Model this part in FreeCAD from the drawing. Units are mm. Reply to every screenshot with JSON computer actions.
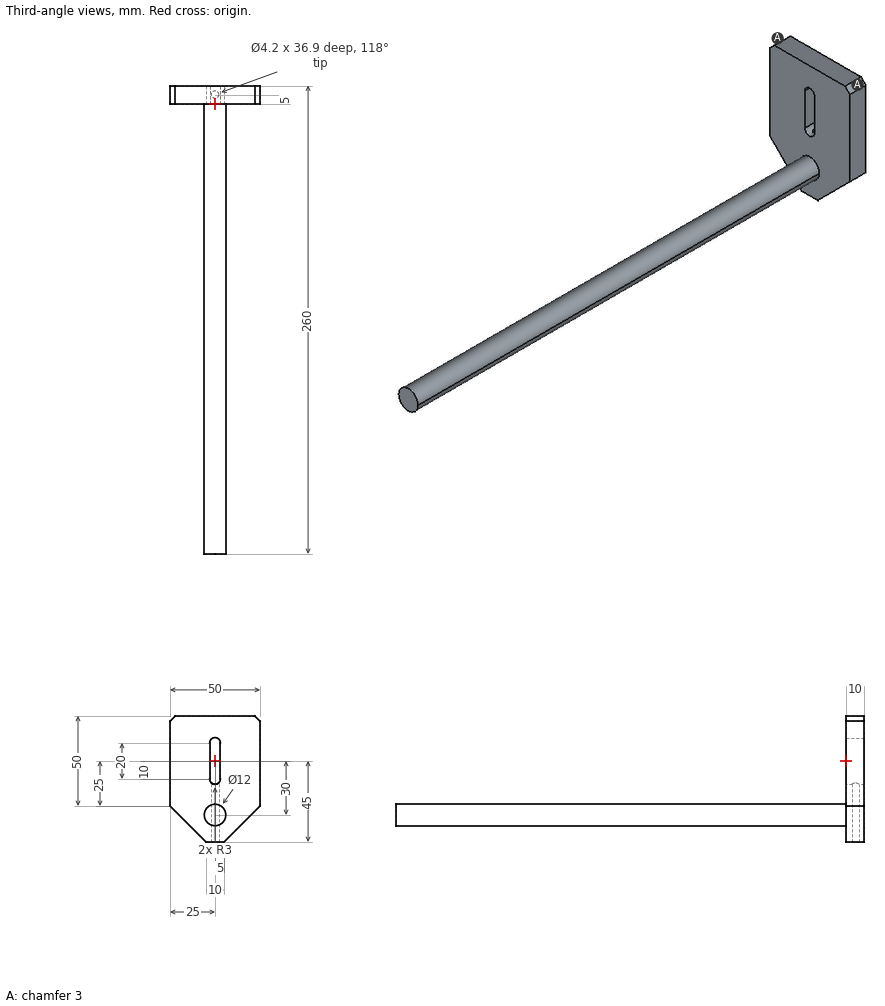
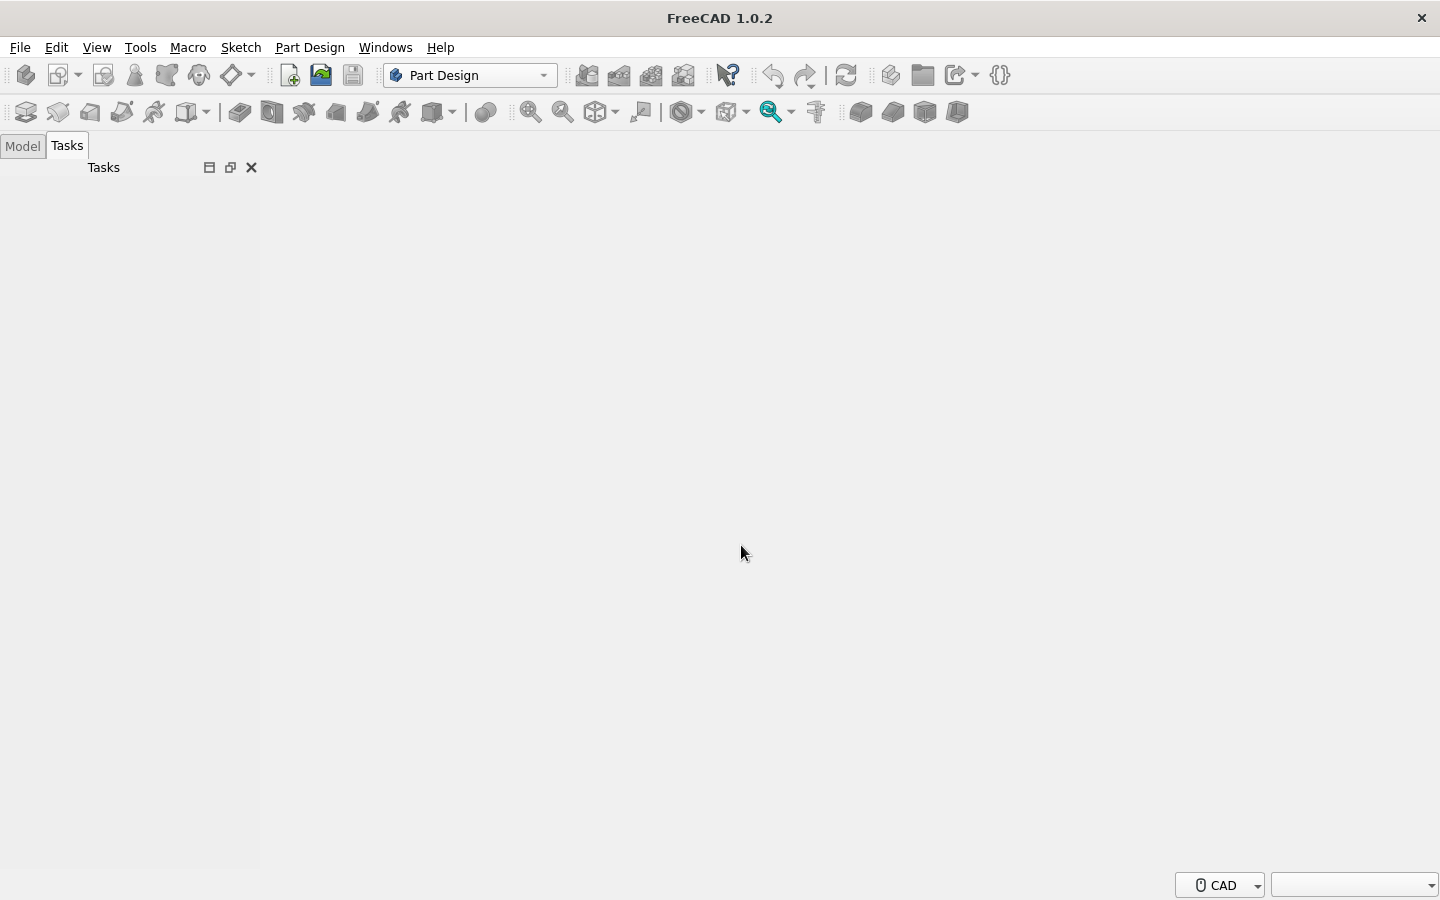
{"action": "left_click", "coordinate": [290, 76]}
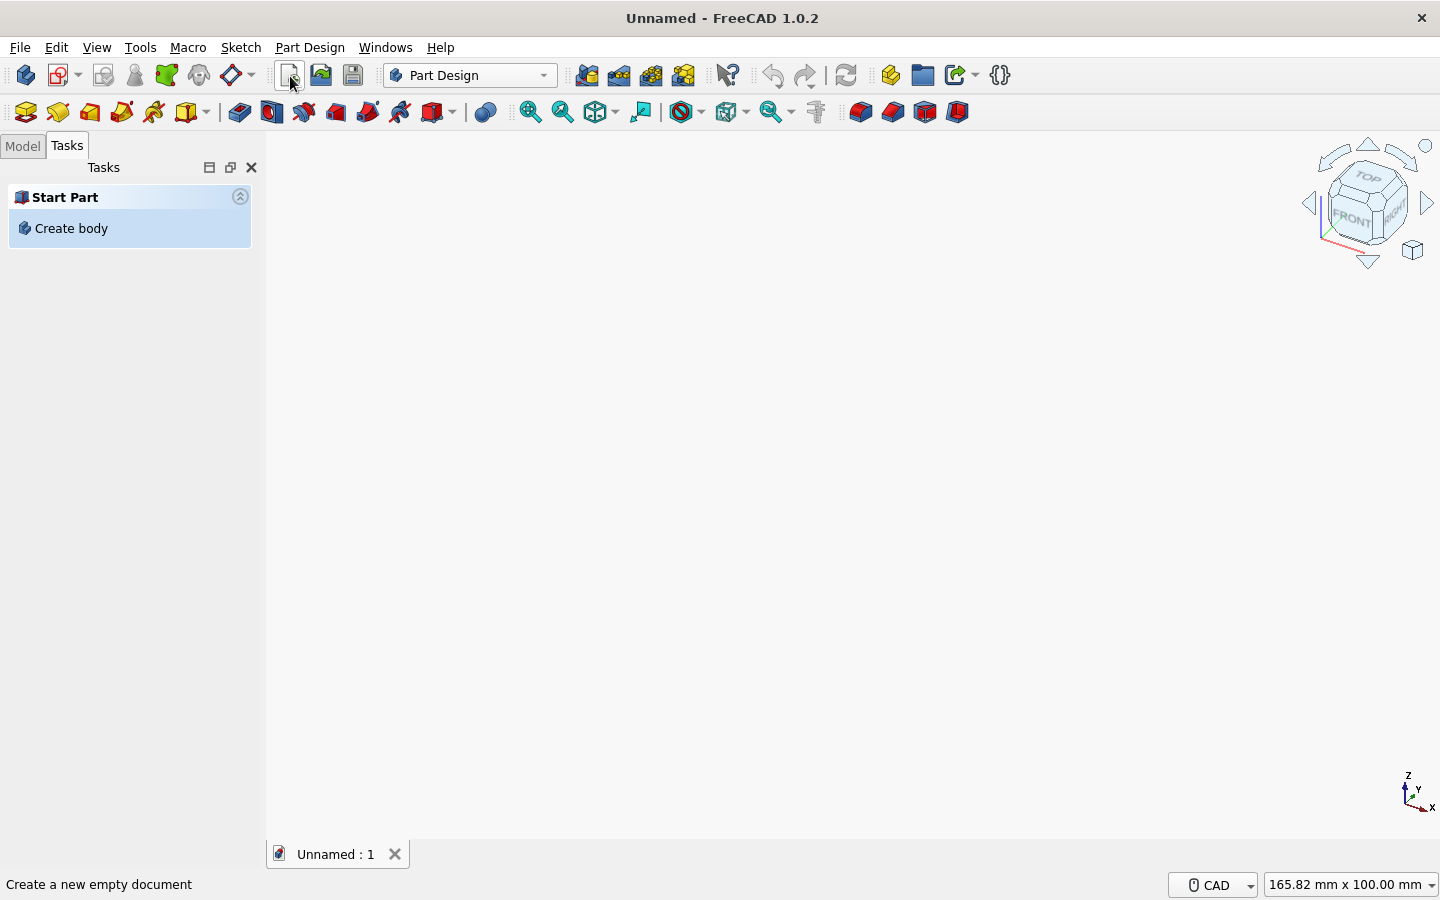
{"action": "left_click", "coordinate": [58, 76]}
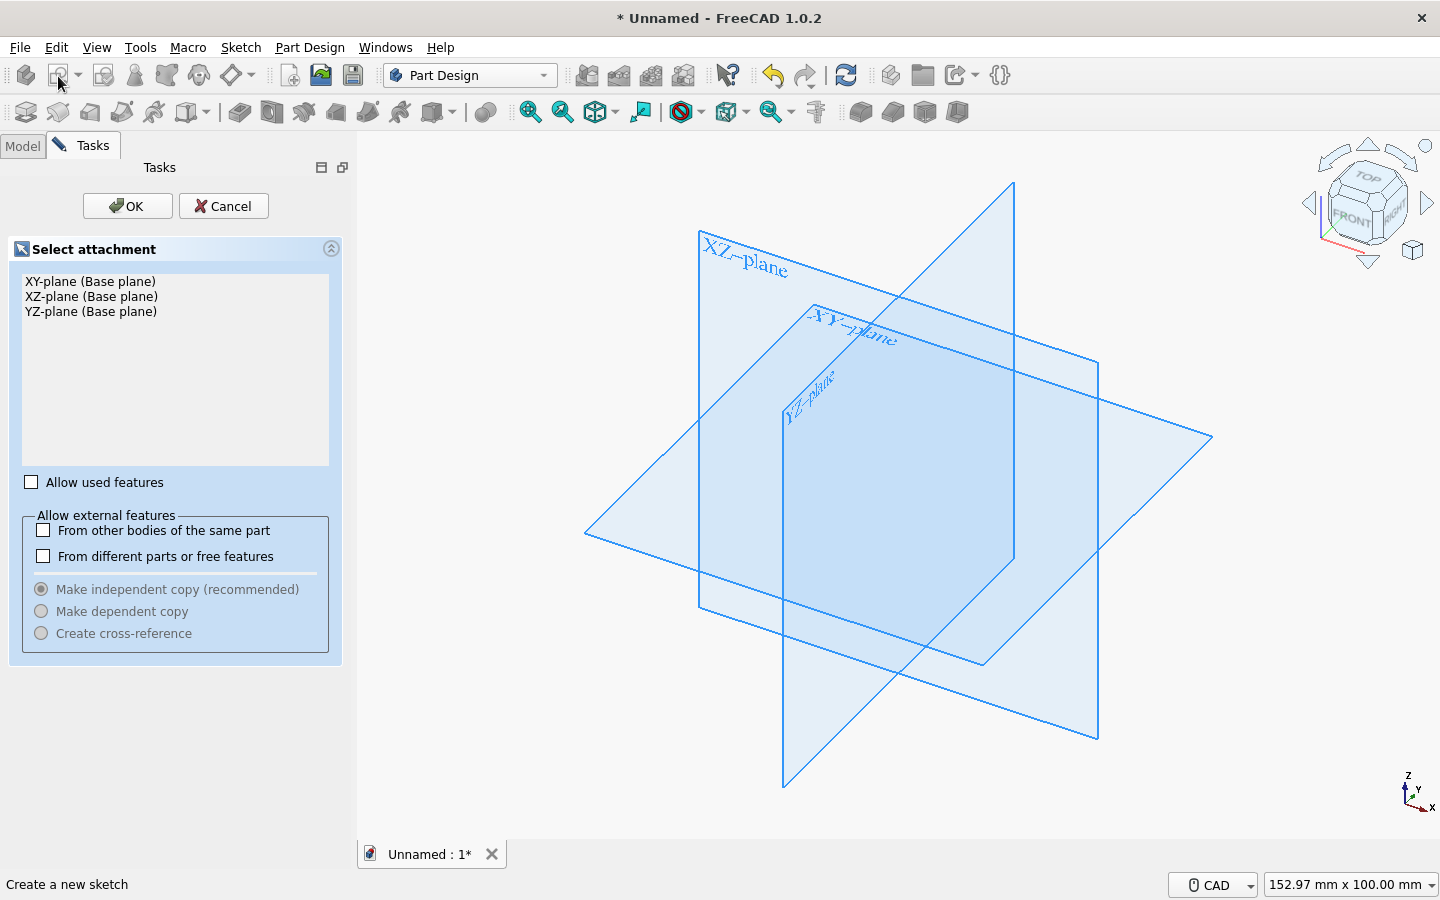
{"action": "left_click", "coordinate": [82, 296]}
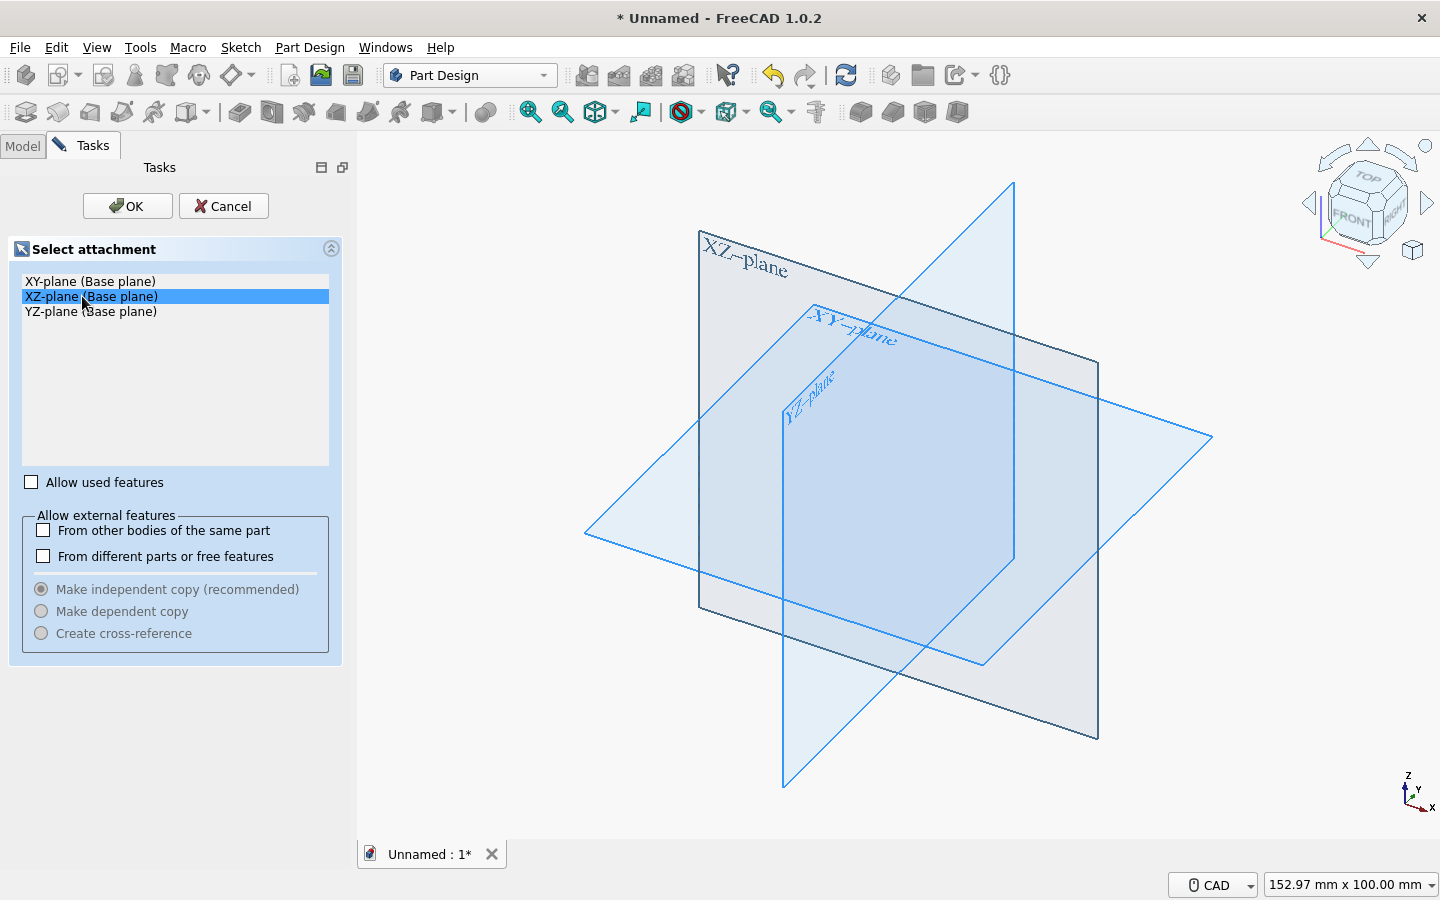
{"action": "left_click", "coordinate": [128, 206]}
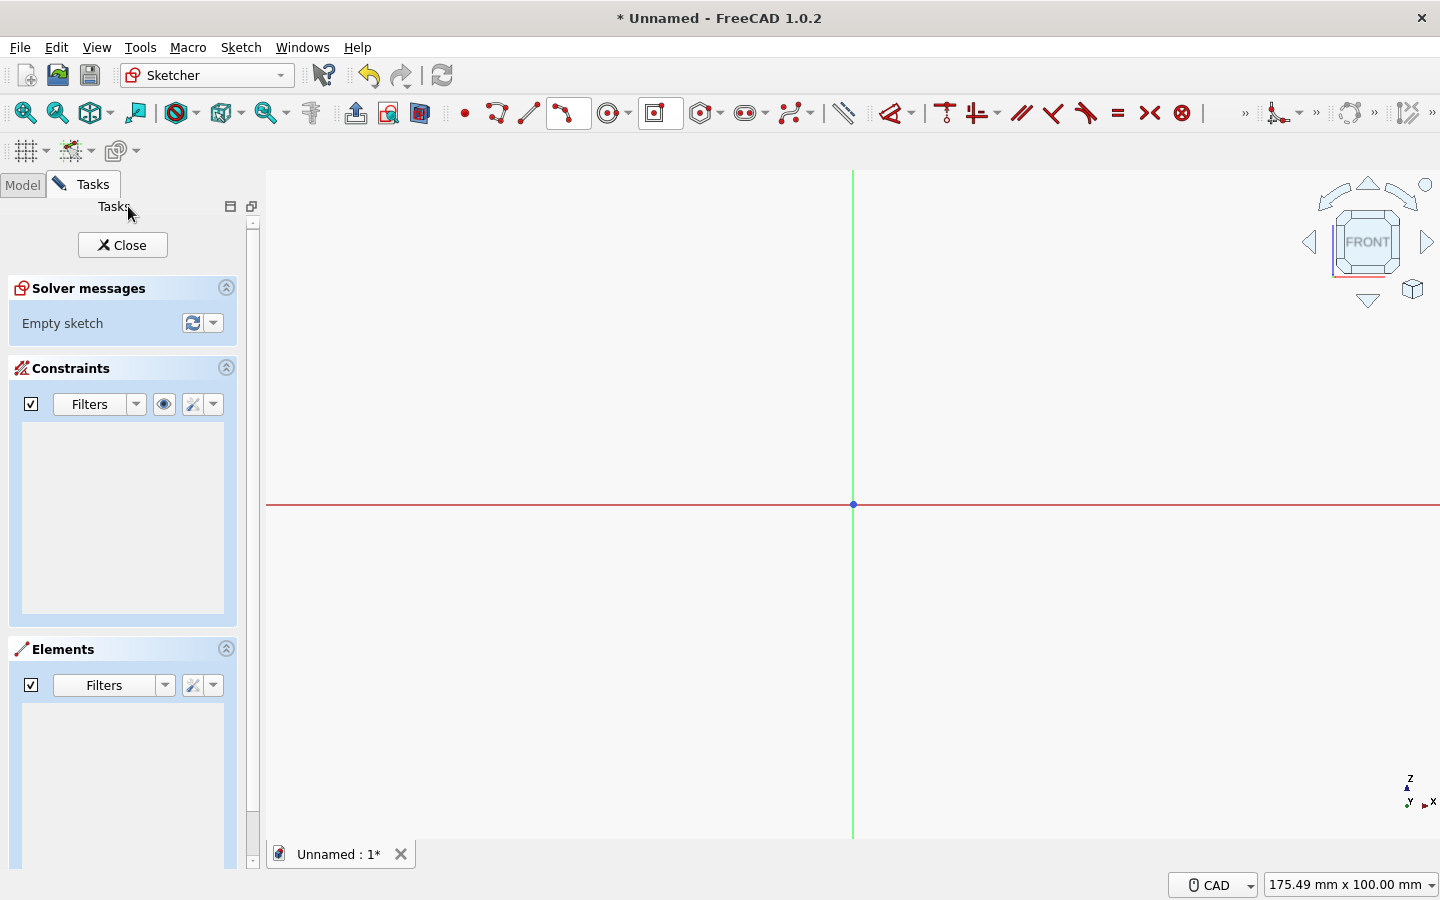
{"action": "scroll", "coordinate": [475, 202], "scroll_direction": "down", "scroll_amount": 1}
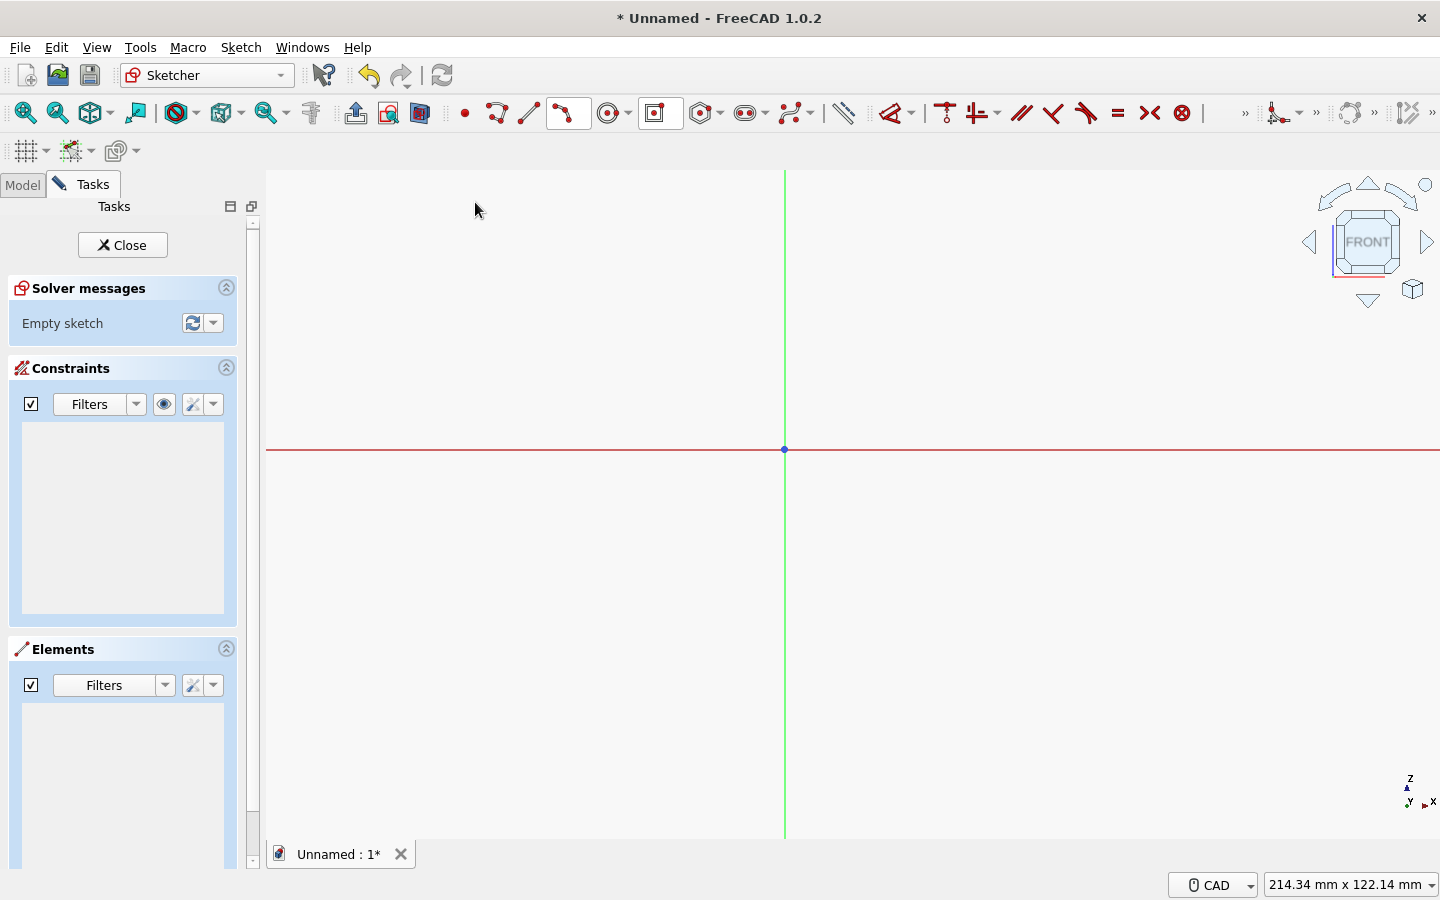
{"action": "left_click", "coordinate": [498, 114]}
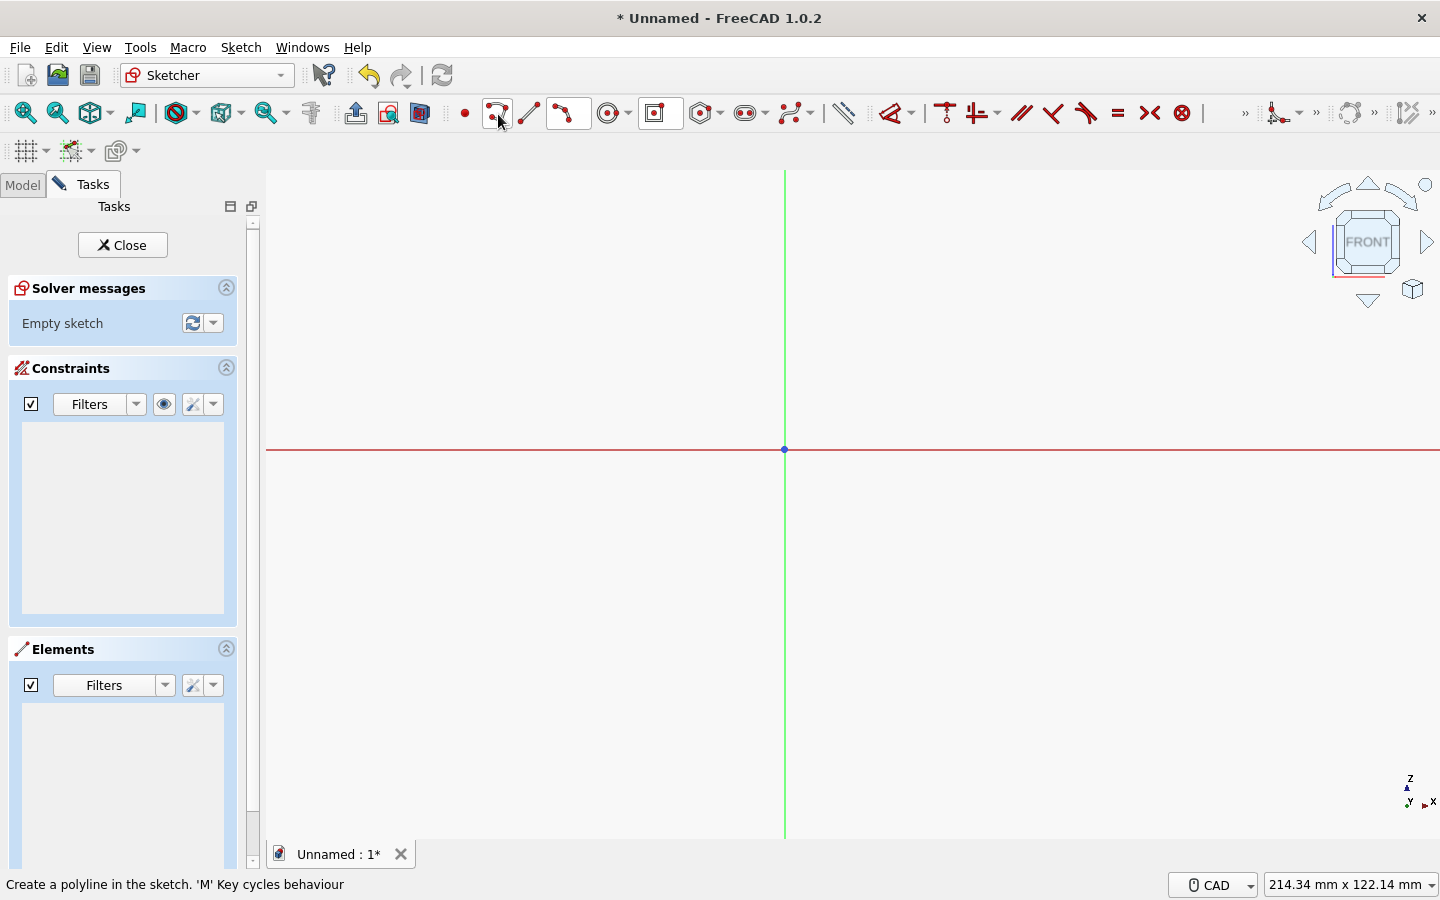
{"action": "left_click", "coordinate": [648, 587]}
{"action": "left_click", "coordinate": [648, 313]}
{"action": "left_click", "coordinate": [921, 313]}
{"action": "left_click", "coordinate": [921, 587]}
{"action": "left_click", "coordinate": [812, 696]}
{"action": "left_click", "coordinate": [757, 696]}
{"action": "left_click", "coordinate": [648, 588]}
{"action": "key", "text": "Escape"}
{"action": "key", "text": "Escape"}